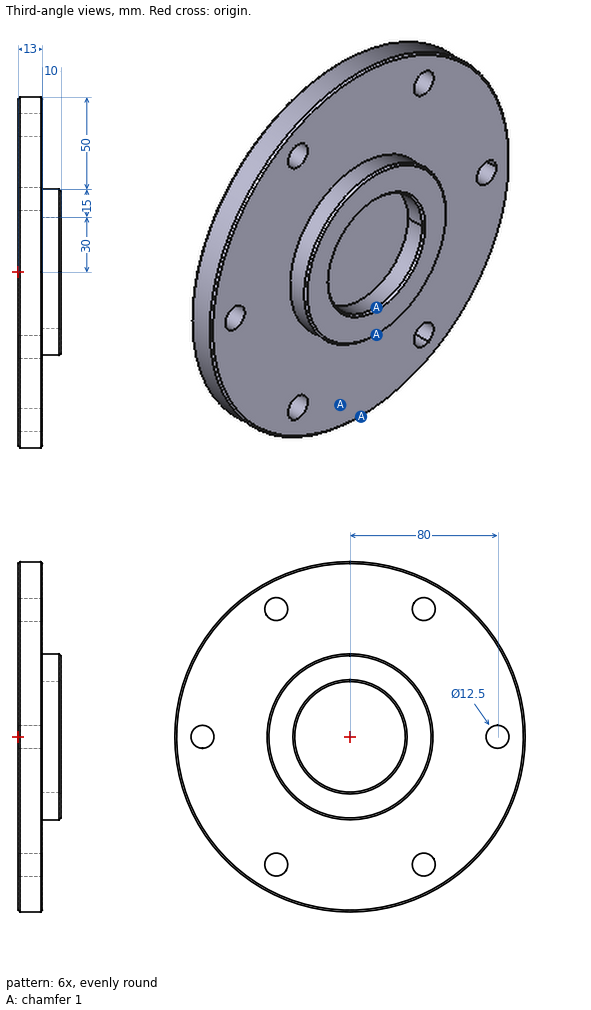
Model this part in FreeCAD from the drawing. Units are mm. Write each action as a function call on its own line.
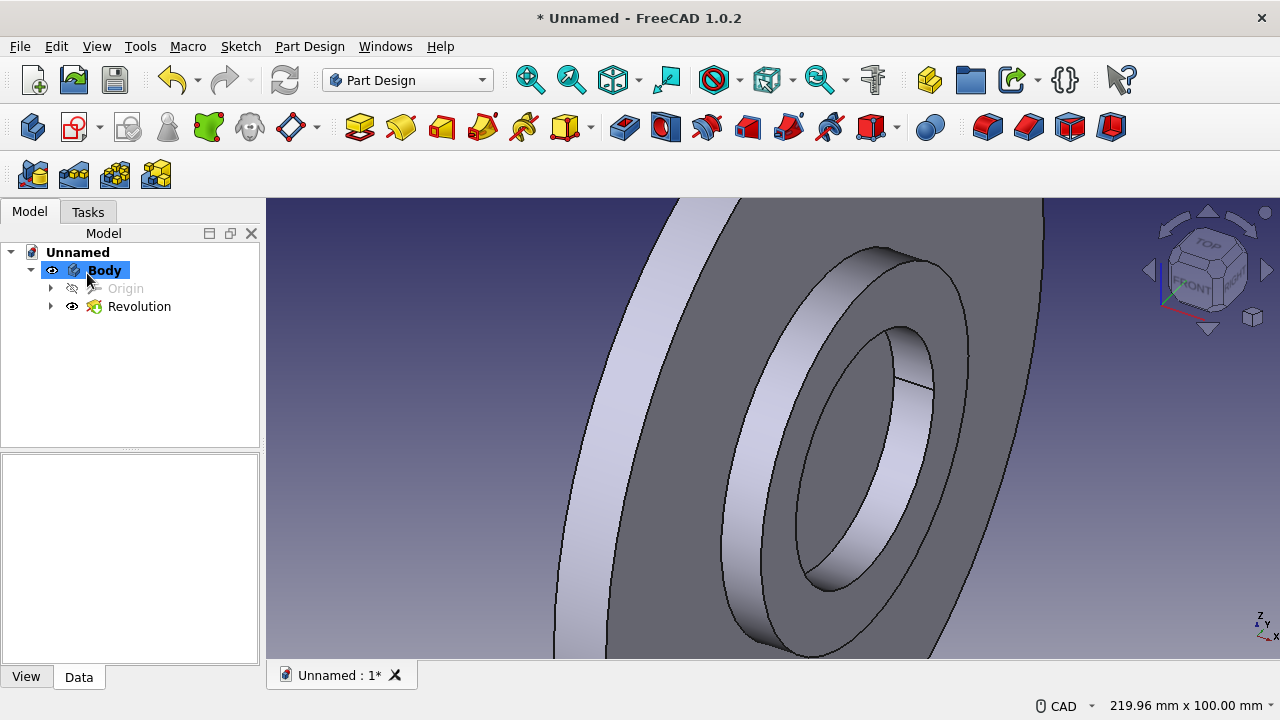
click(531, 80)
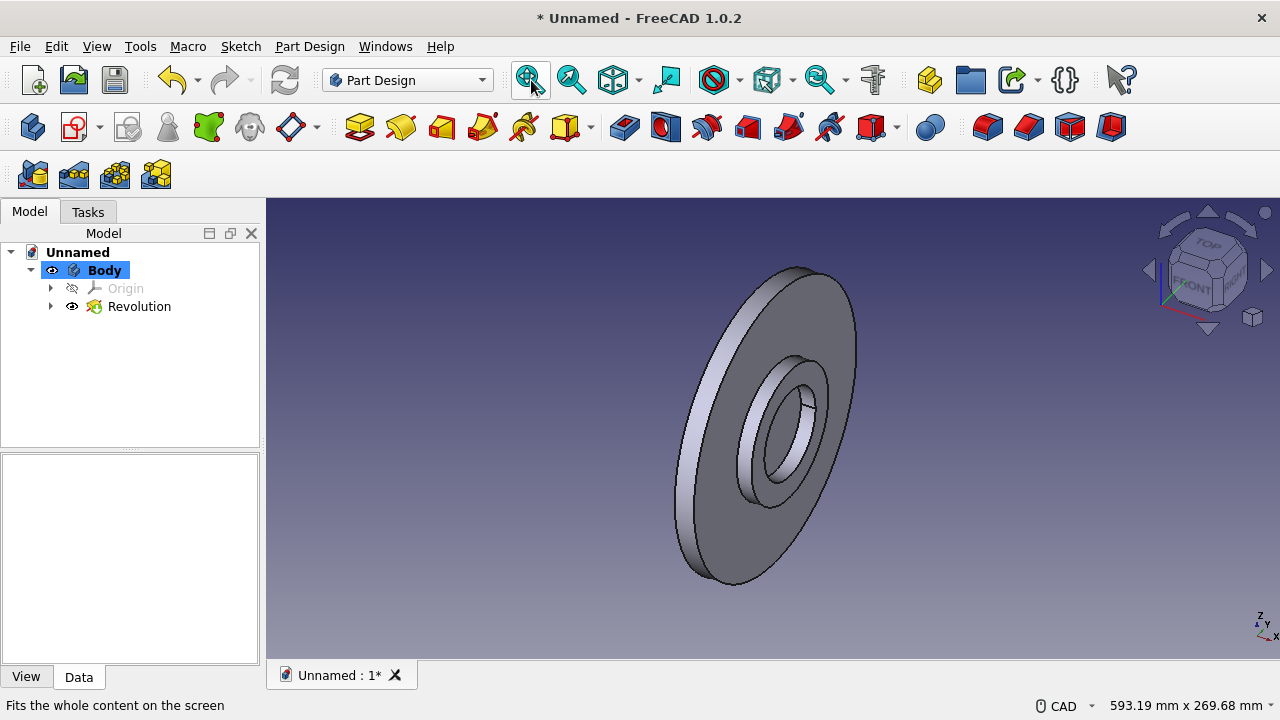
click(74, 128)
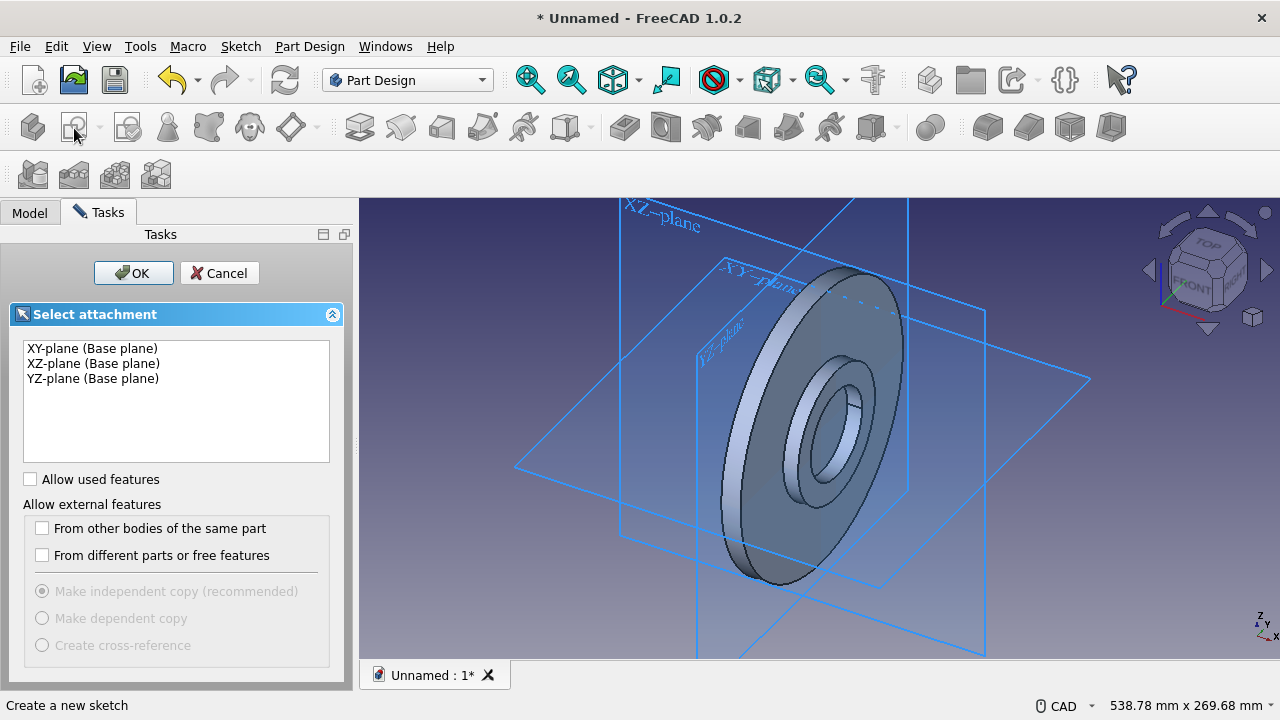
click(84, 378)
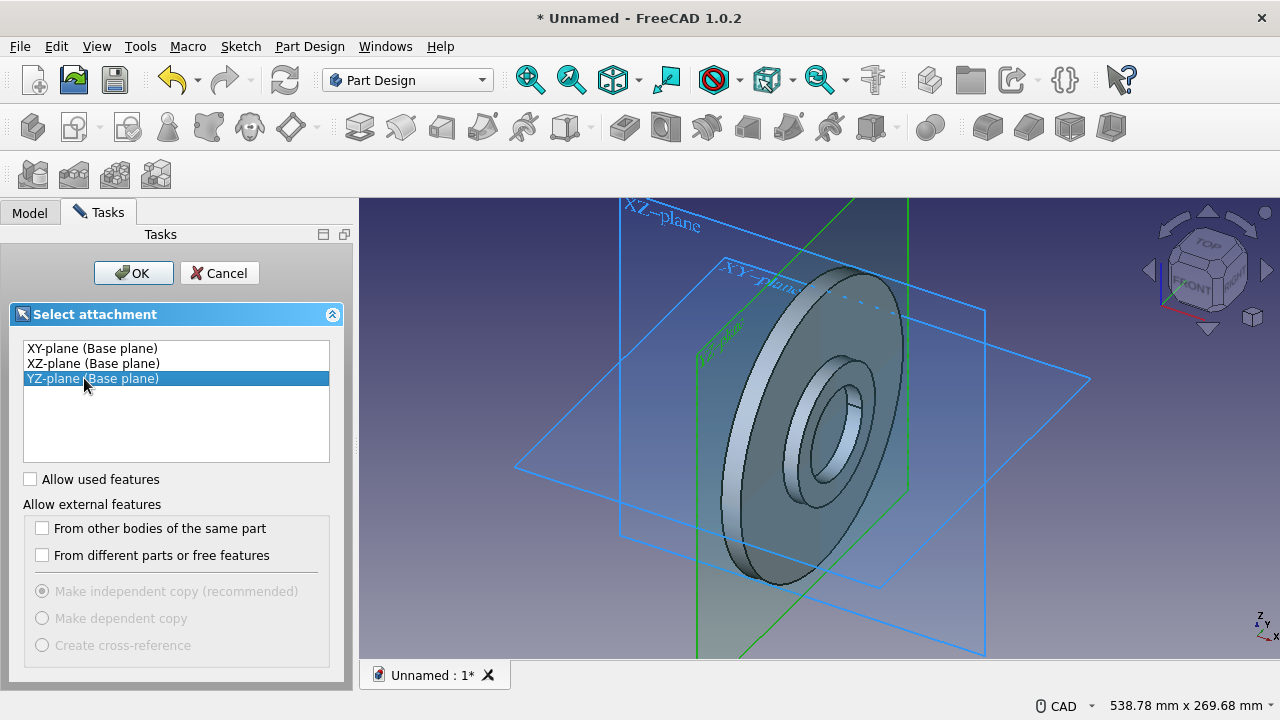
click(134, 273)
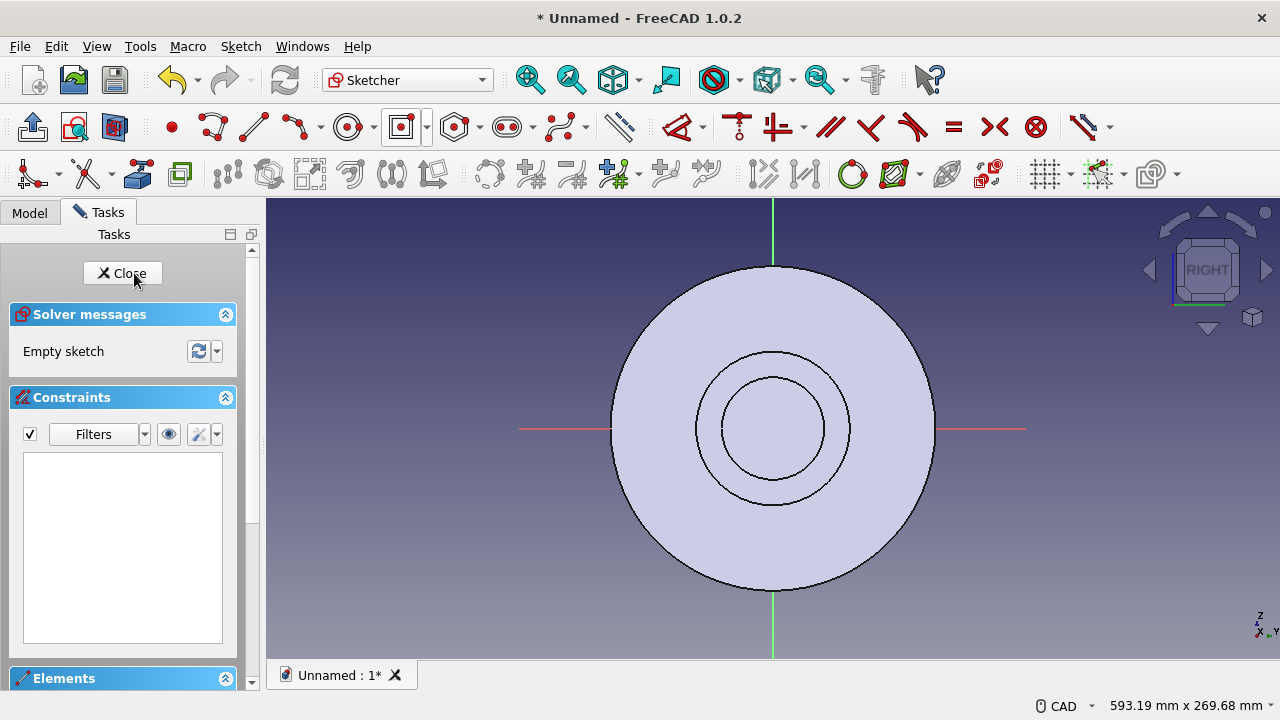
click(115, 128)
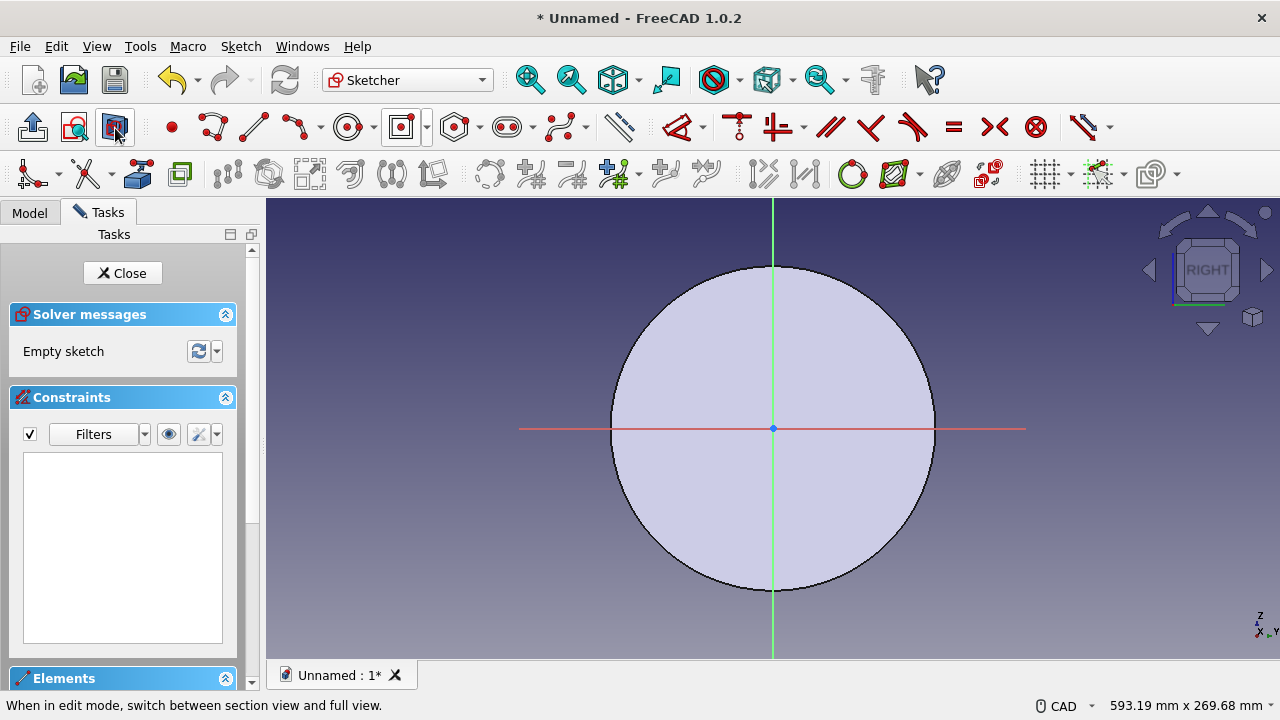
scroll(926, 428, up, 13)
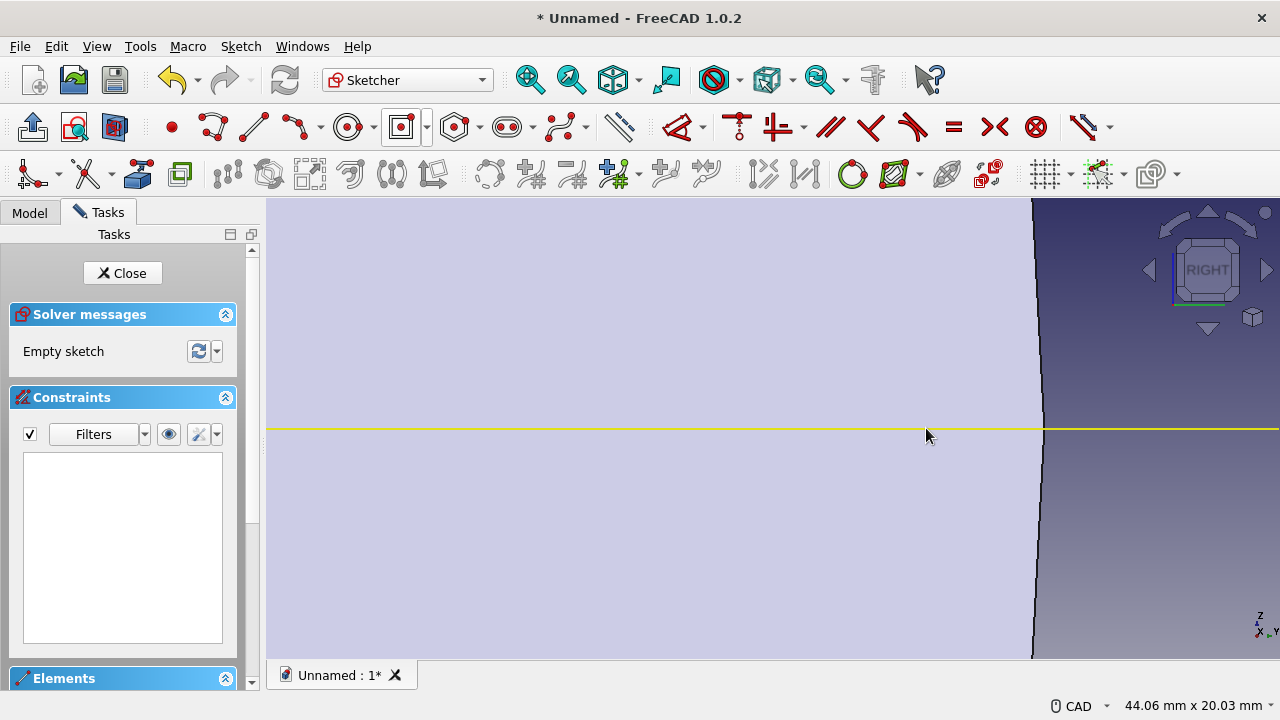
key(g)
key(c)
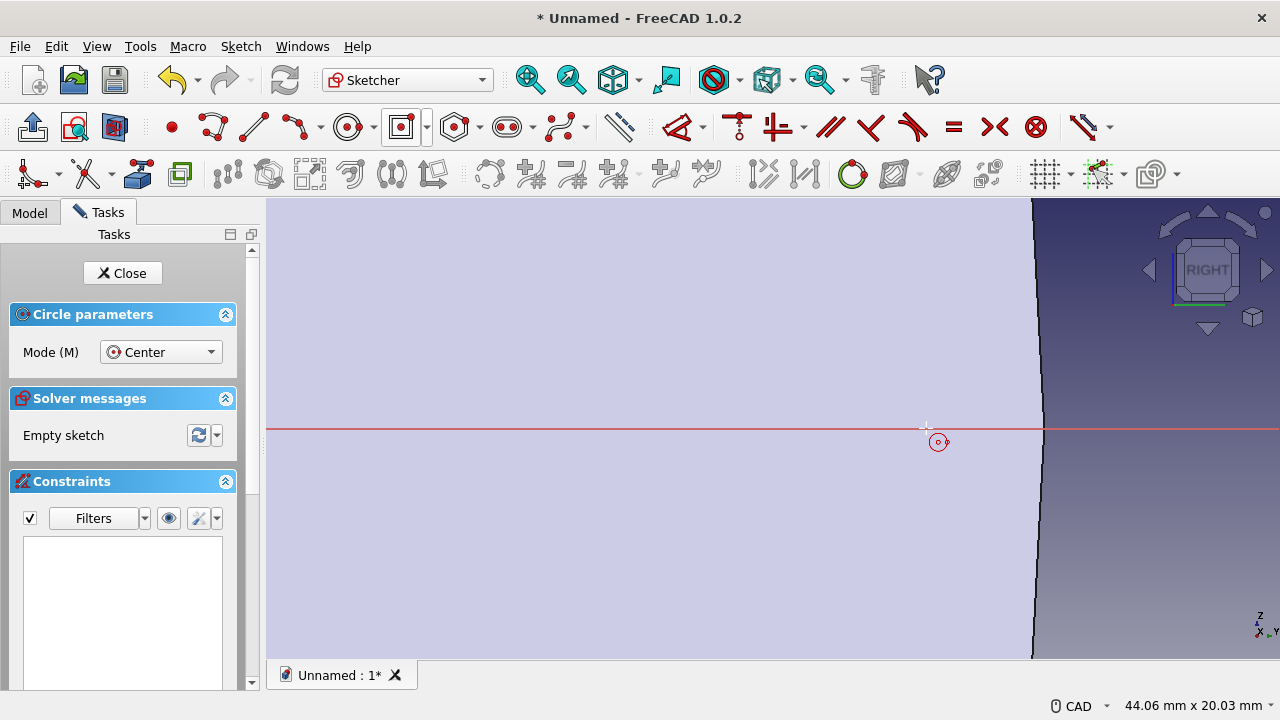
click(699, 428)
click(801, 327)
key(Escape)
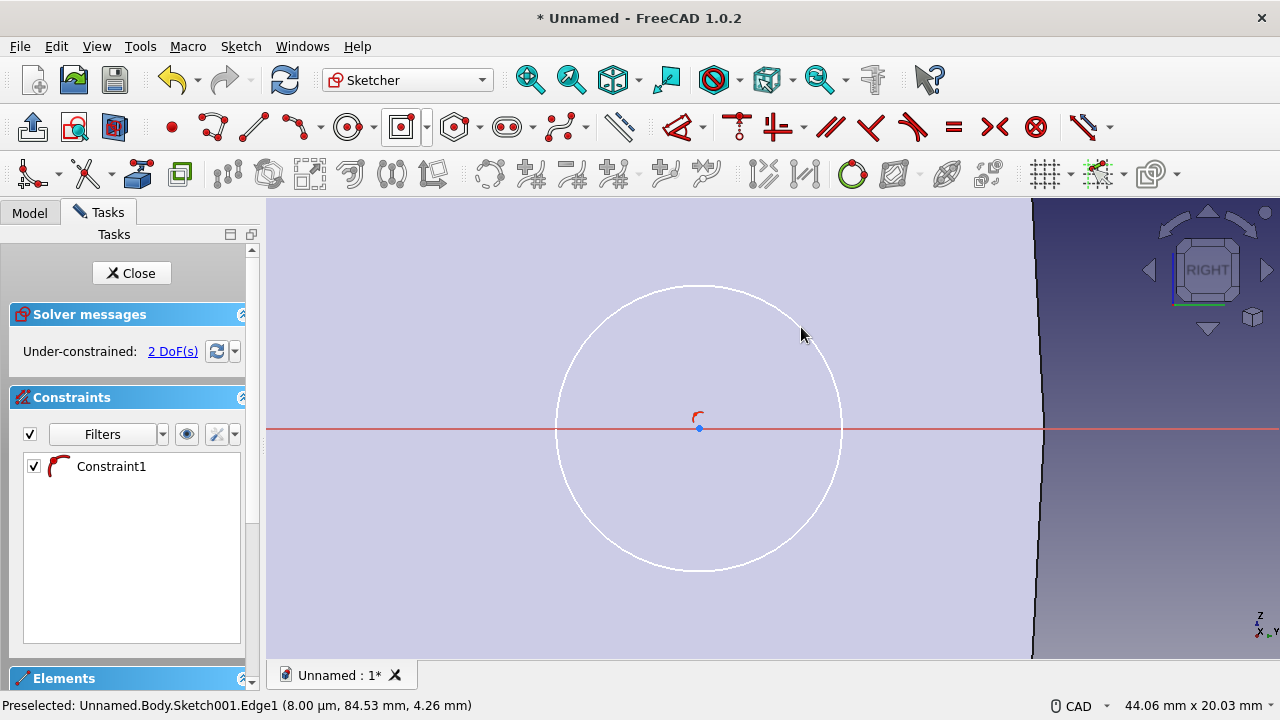
key(d)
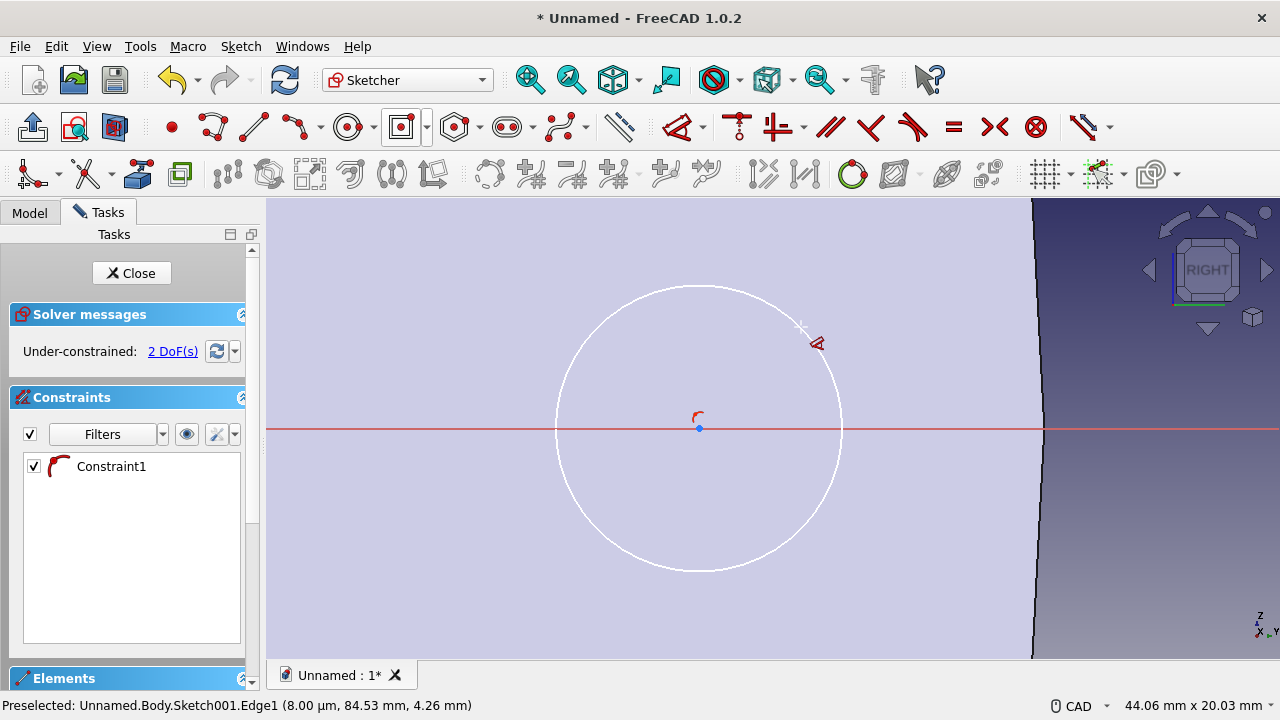
click(800, 327)
click(823, 304)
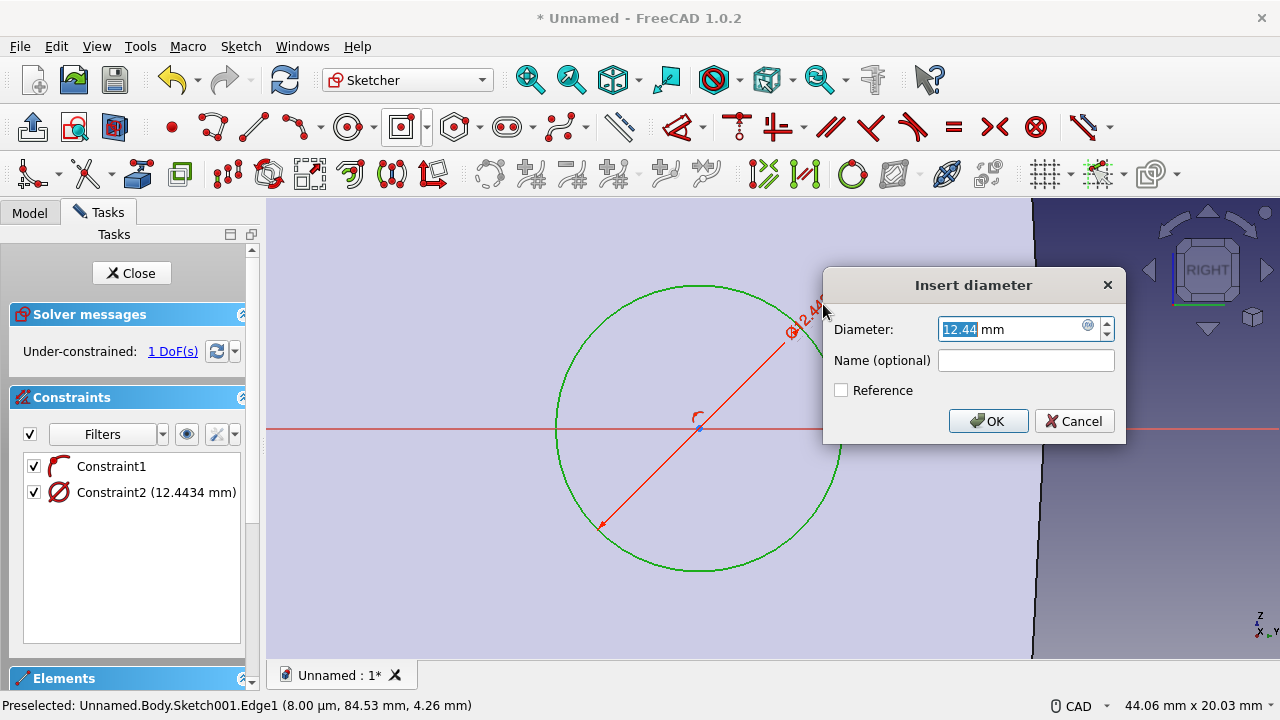
text(12.5)
key(Return)